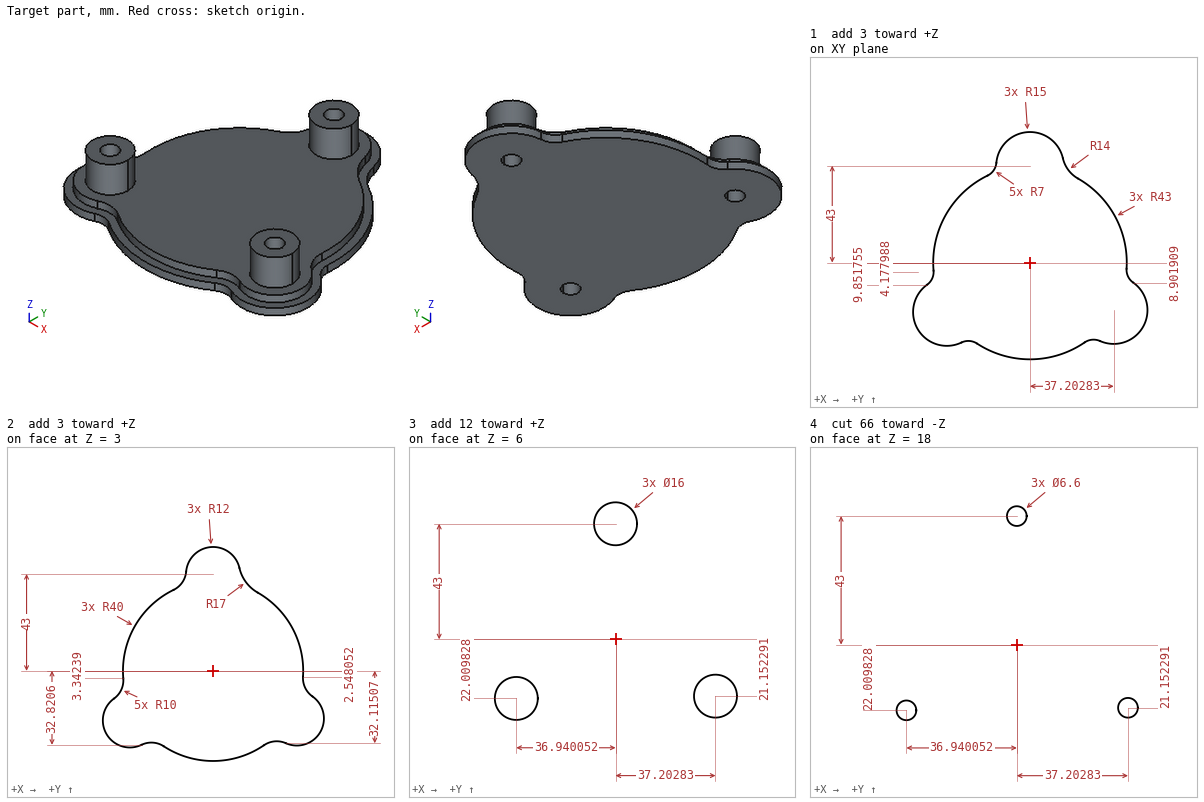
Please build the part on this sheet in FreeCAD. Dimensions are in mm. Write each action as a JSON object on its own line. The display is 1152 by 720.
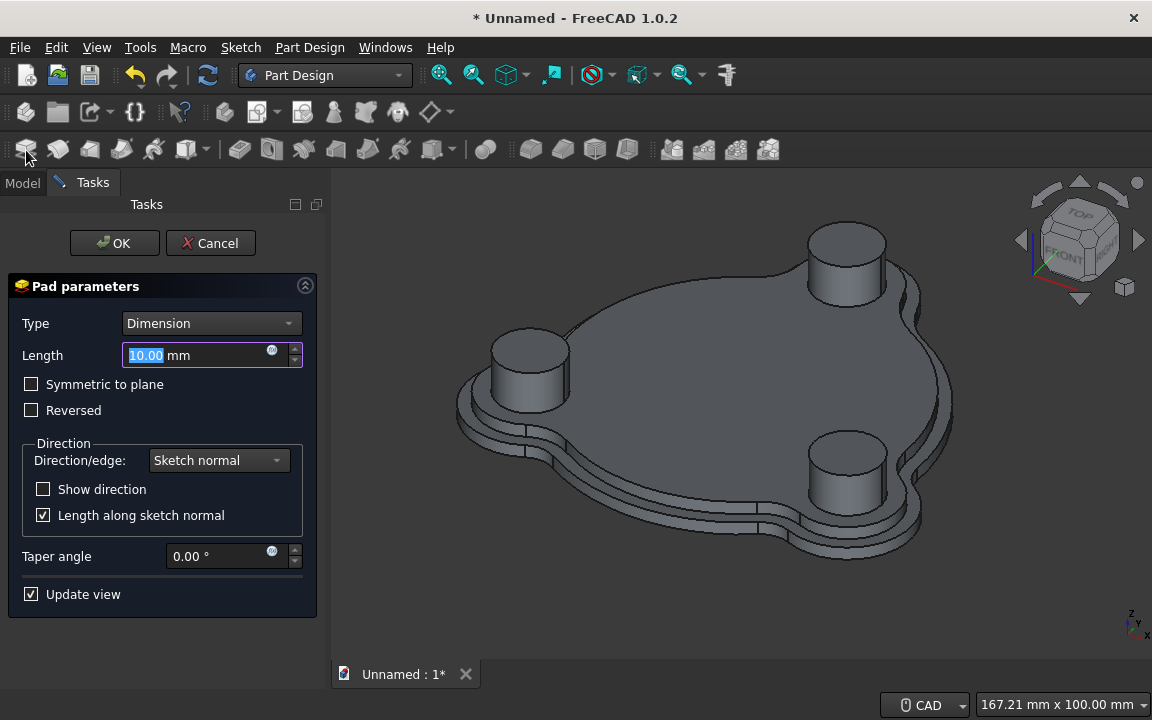
{"action": "type", "text": "12"}
{"action": "key", "text": "Tab"}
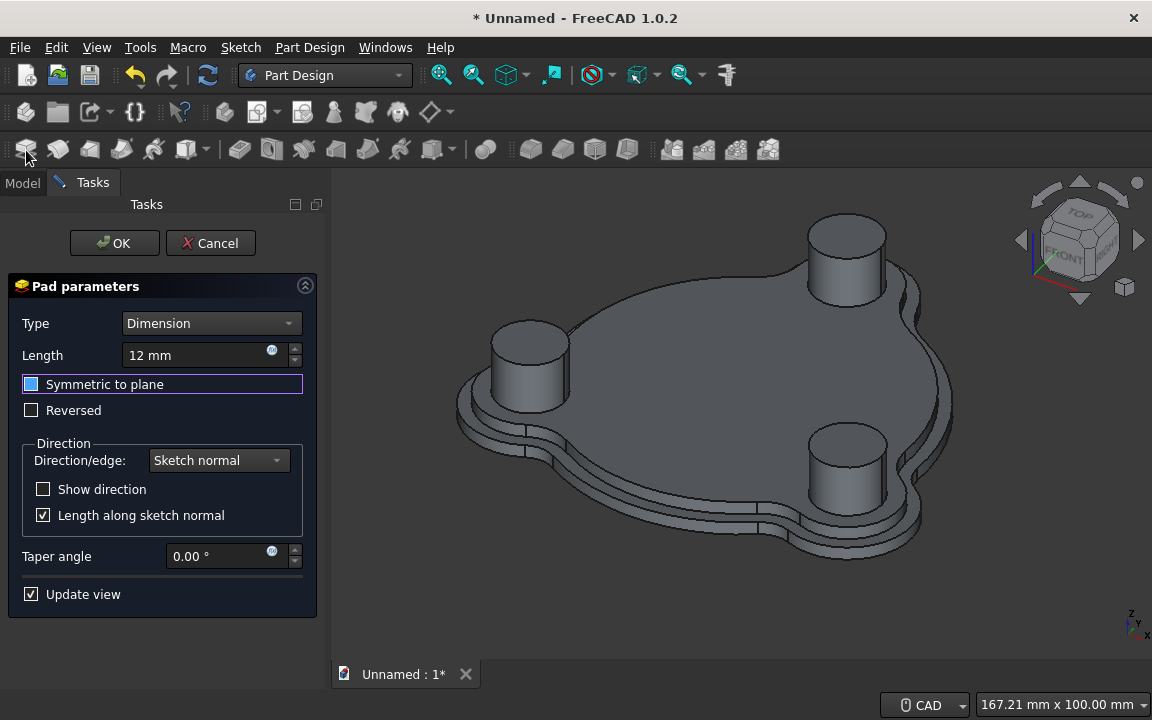
{"action": "left_click", "coordinate": [115, 243]}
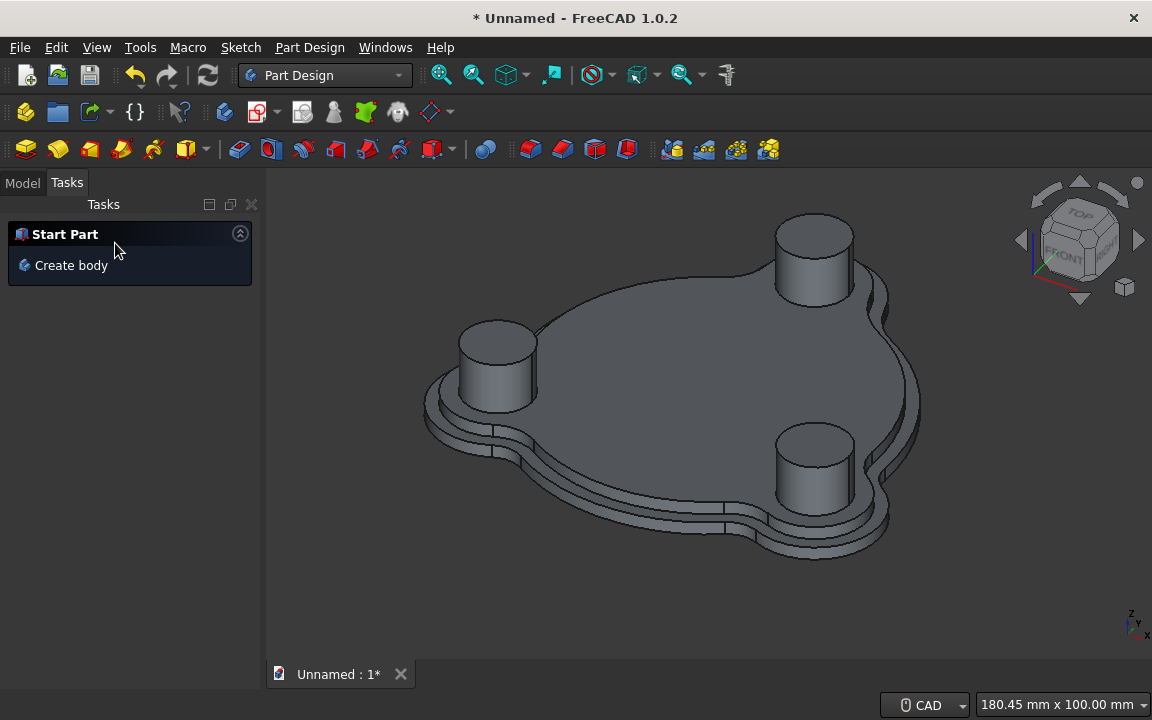
{"action": "left_click", "coordinate": [442, 76]}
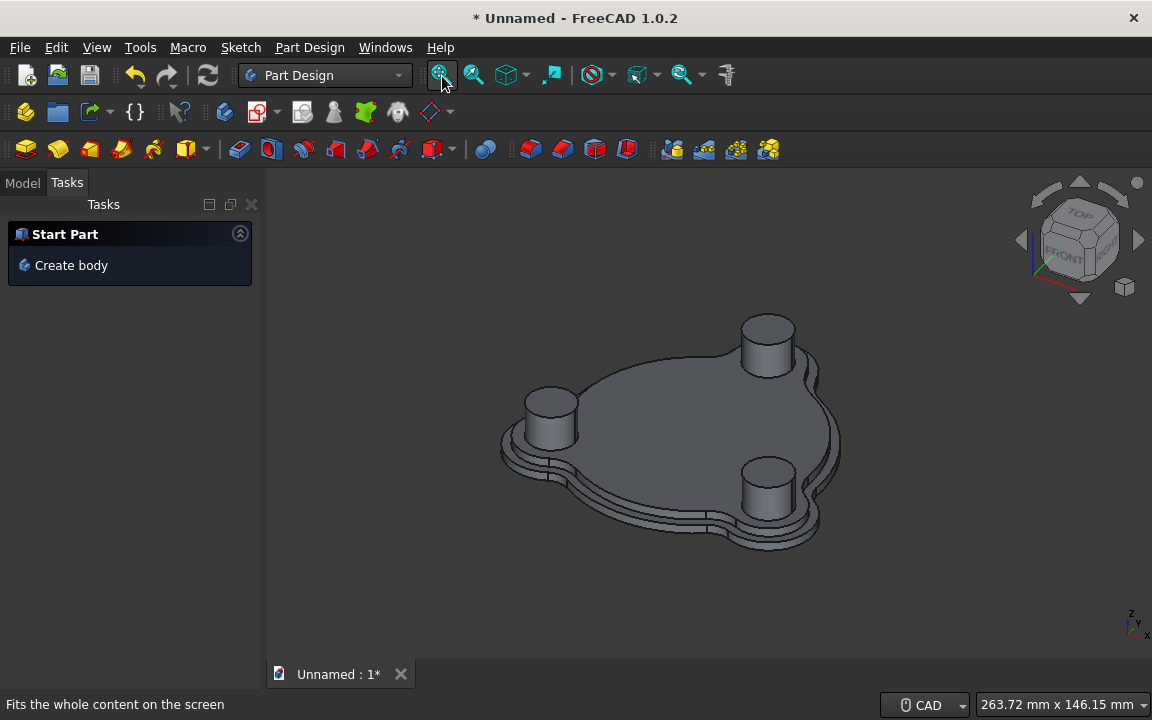
{"action": "left_click", "coordinate": [769, 471]}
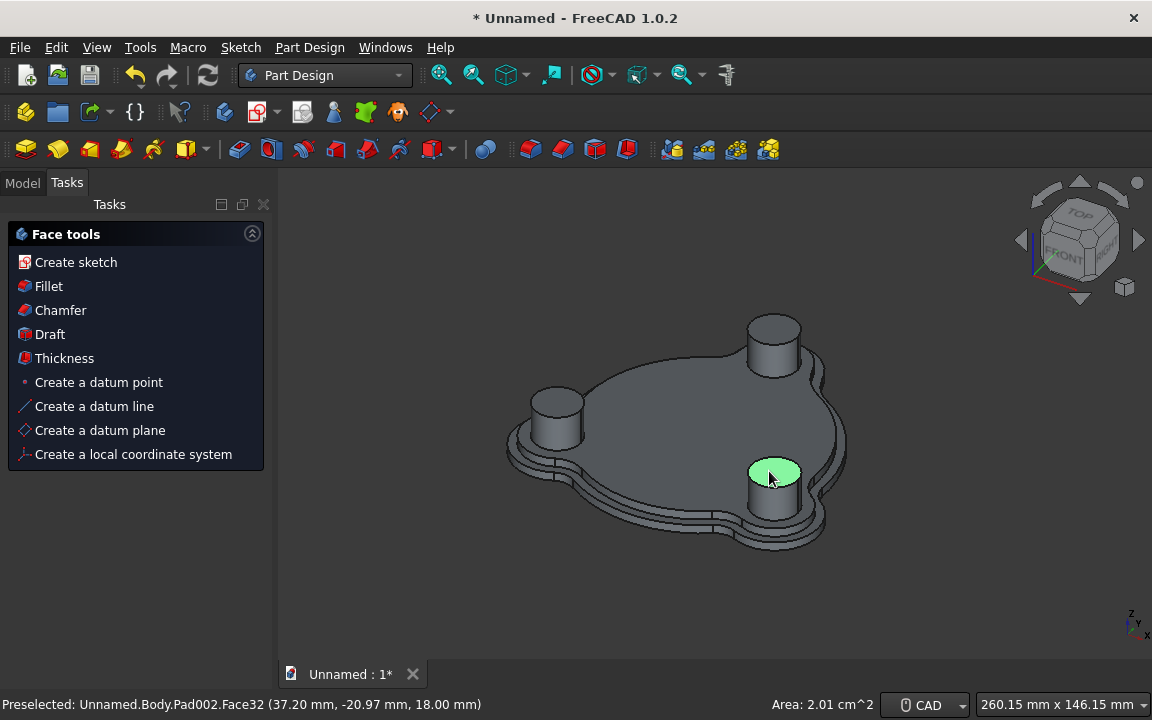
{"action": "left_click", "coordinate": [258, 112]}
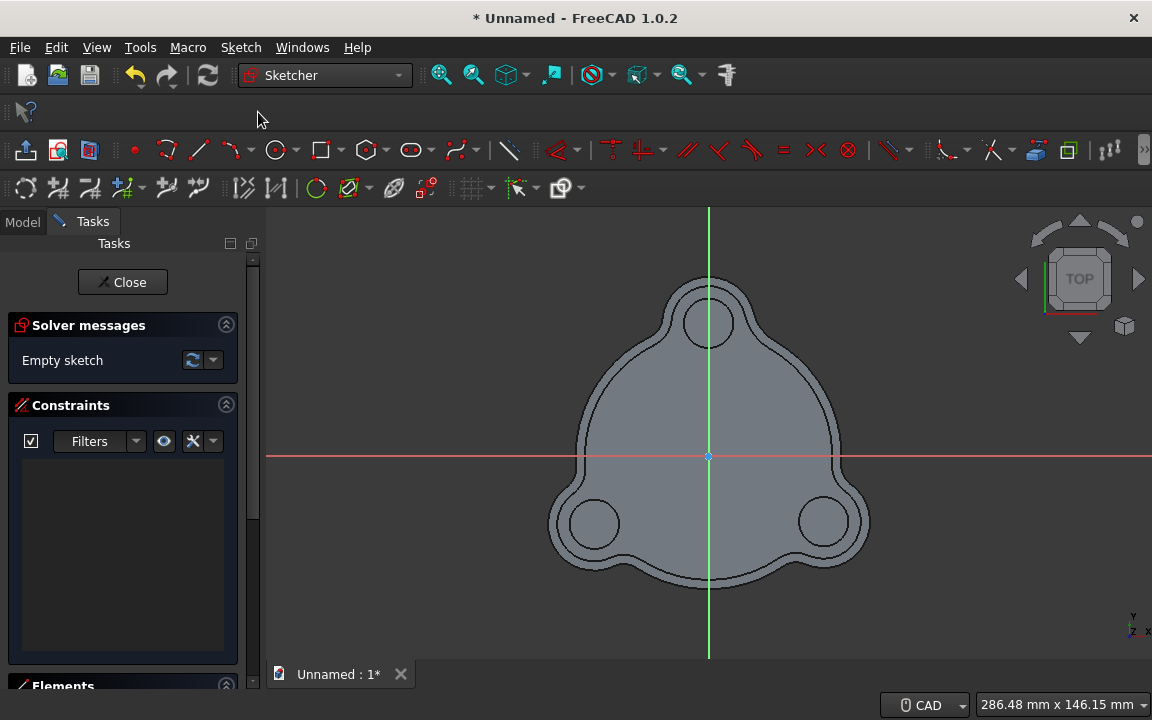
{"action": "left_click", "coordinate": [276, 150]}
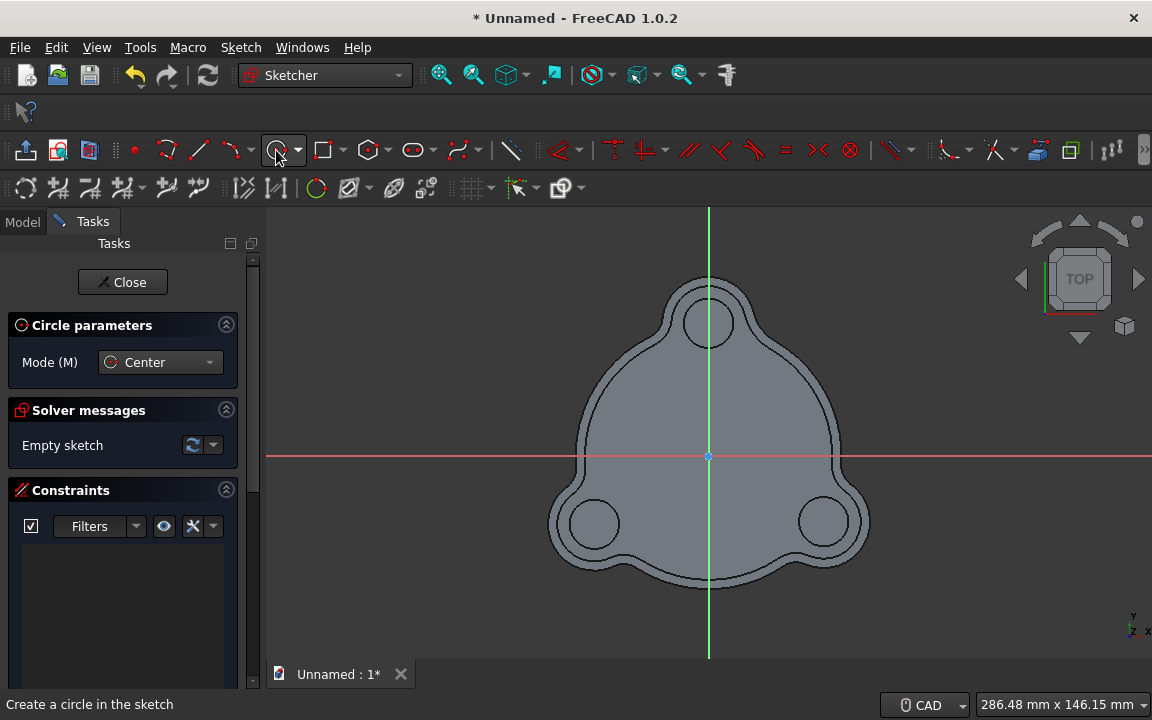
{"action": "scroll", "coordinate": [709, 323], "scroll_direction": "up", "scroll_amount": 4}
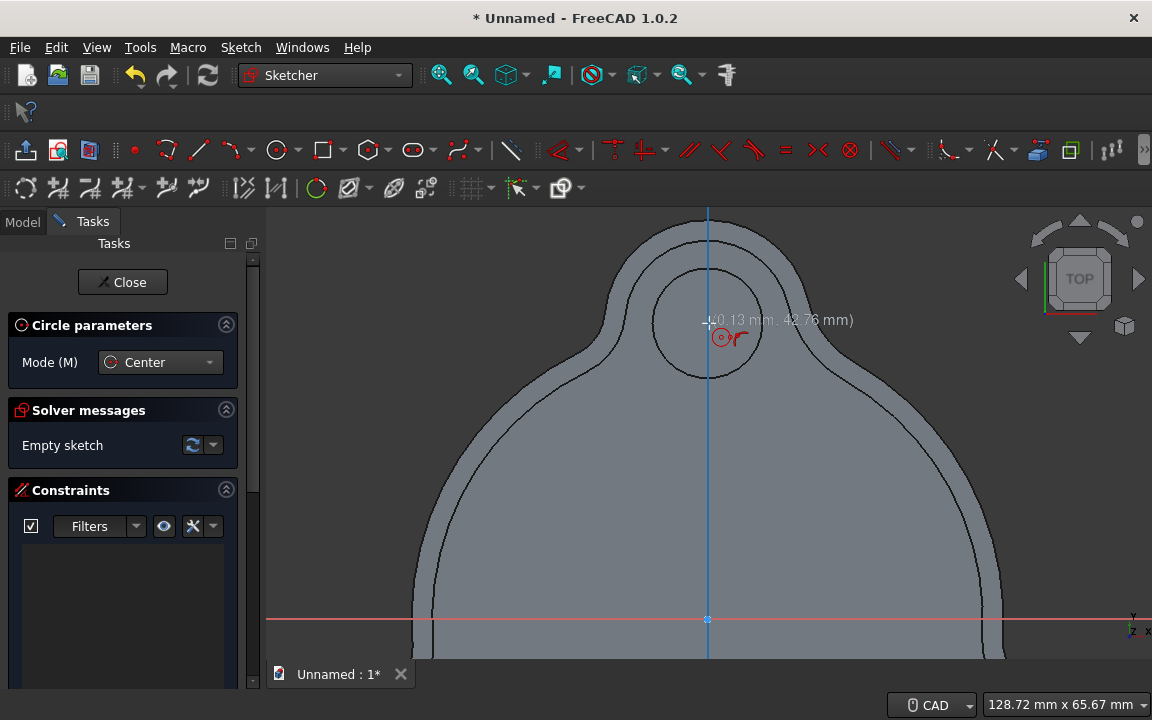
{"action": "left_click", "coordinate": [708, 323]}
{"action": "left_click", "coordinate": [724, 307]}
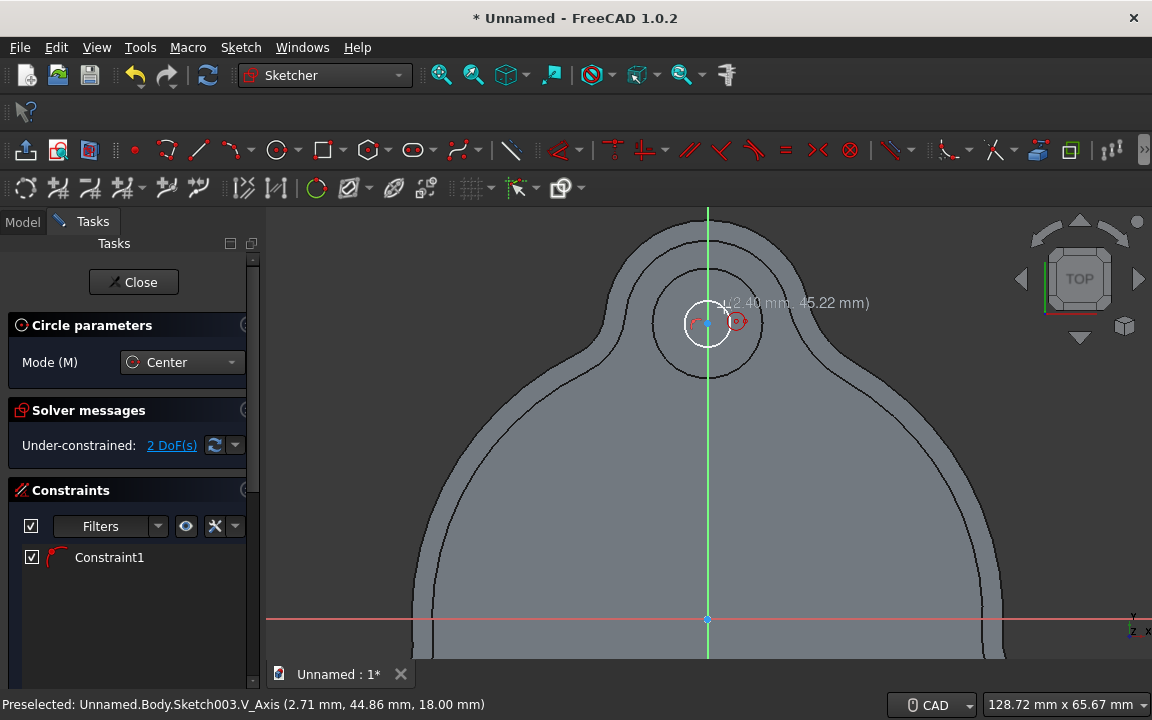
{"action": "scroll", "coordinate": [558, 294], "scroll_direction": "down", "scroll_amount": 3}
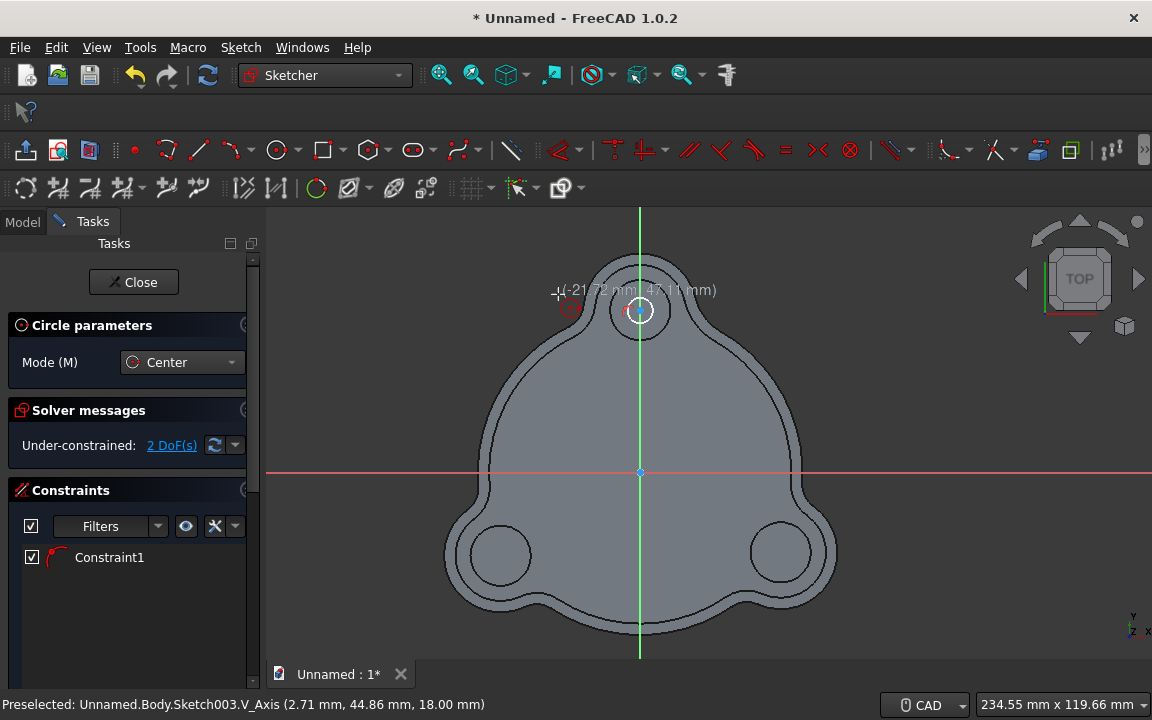
{"action": "scroll", "coordinate": [781, 552], "scroll_direction": "up", "scroll_amount": 3}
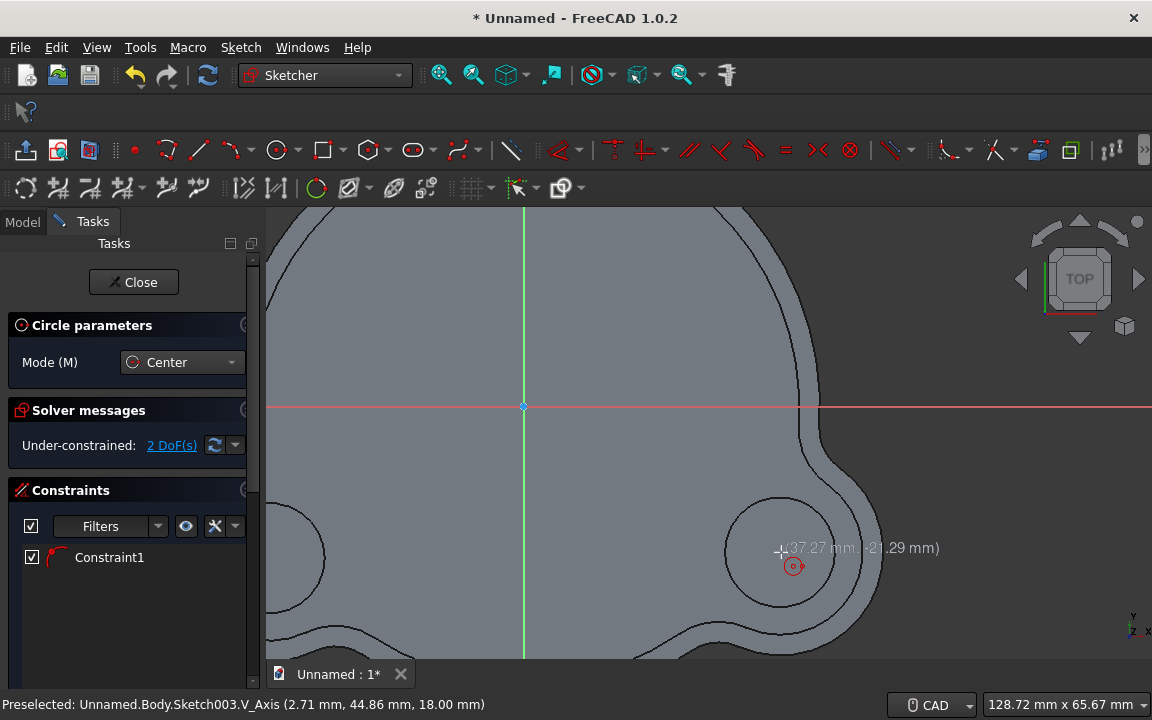
{"action": "left_click", "coordinate": [780, 552]}
{"action": "left_click", "coordinate": [796, 536]}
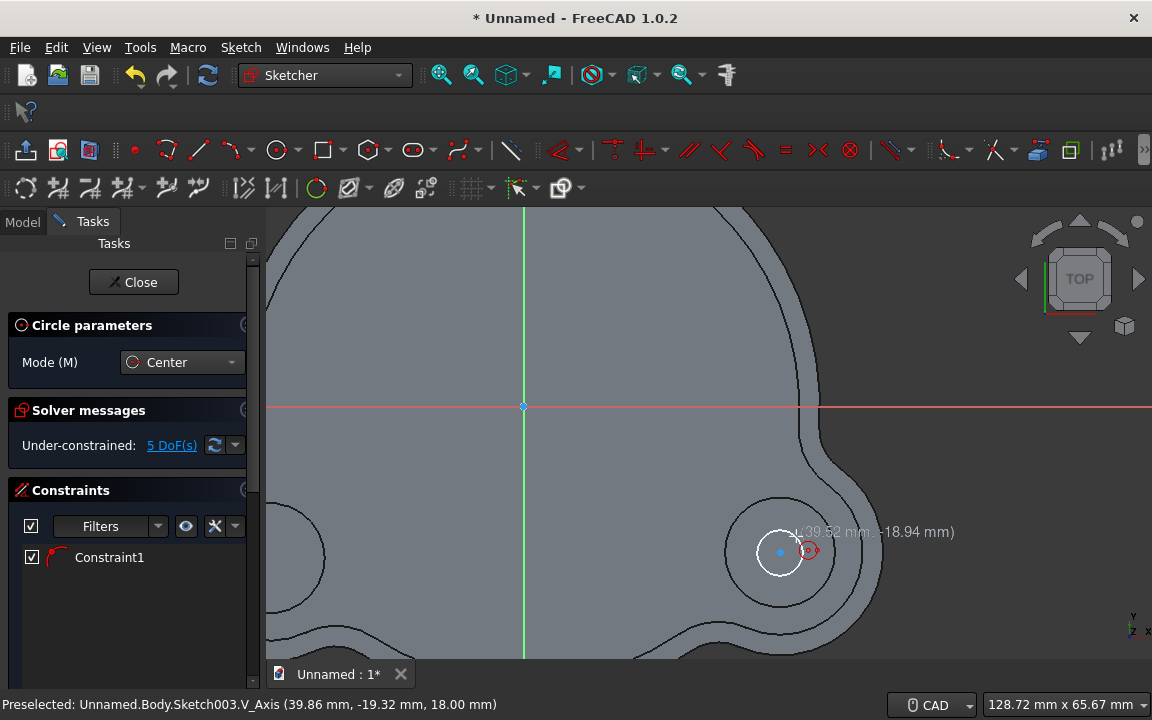
{"action": "scroll", "coordinate": [781, 553], "scroll_direction": "down", "scroll_amount": 3}